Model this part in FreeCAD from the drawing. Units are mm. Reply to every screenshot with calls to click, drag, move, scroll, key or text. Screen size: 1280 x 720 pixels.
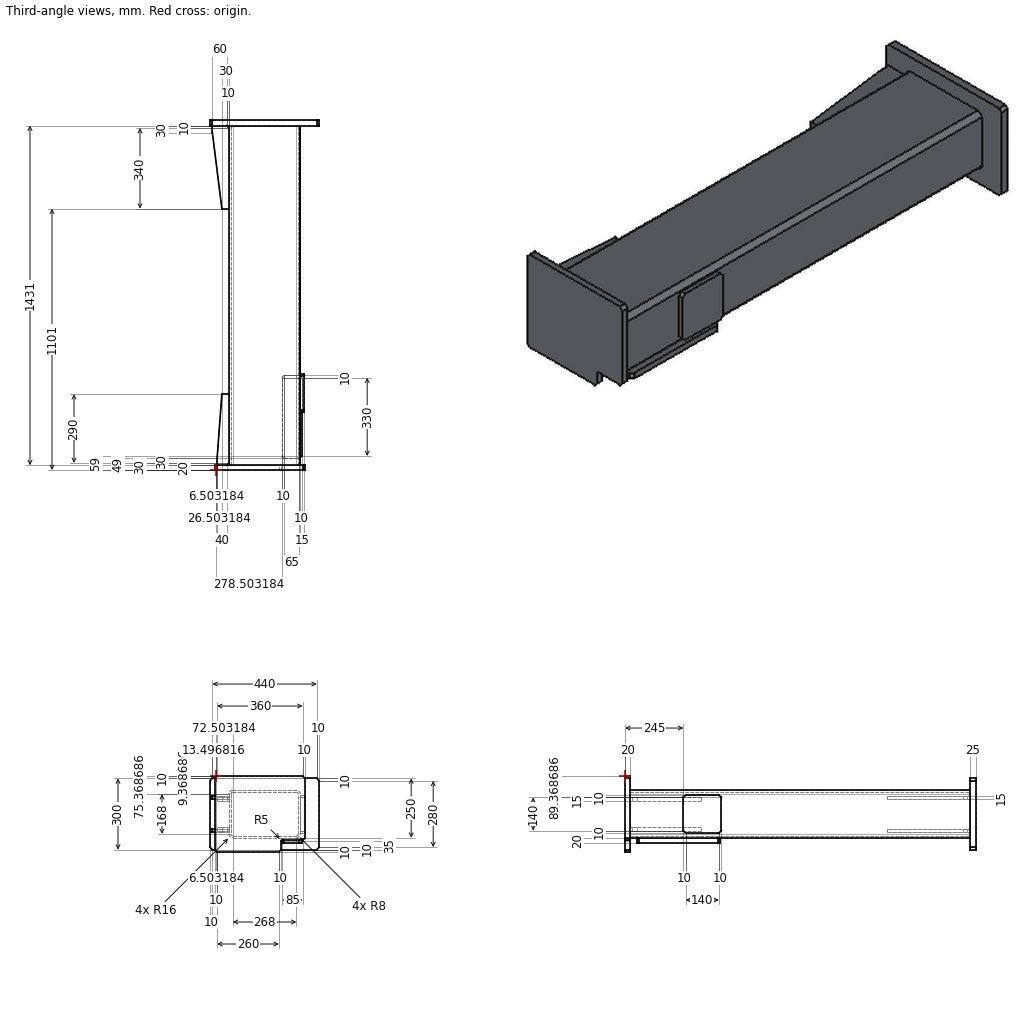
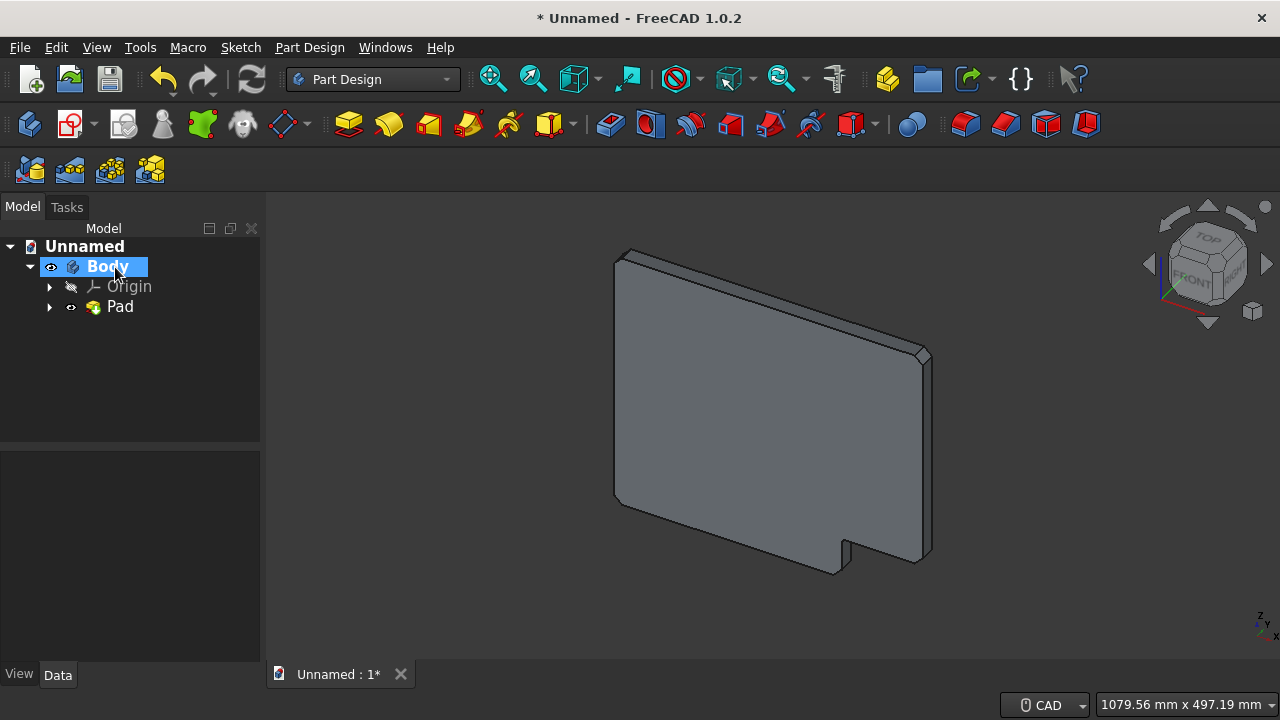
key(4)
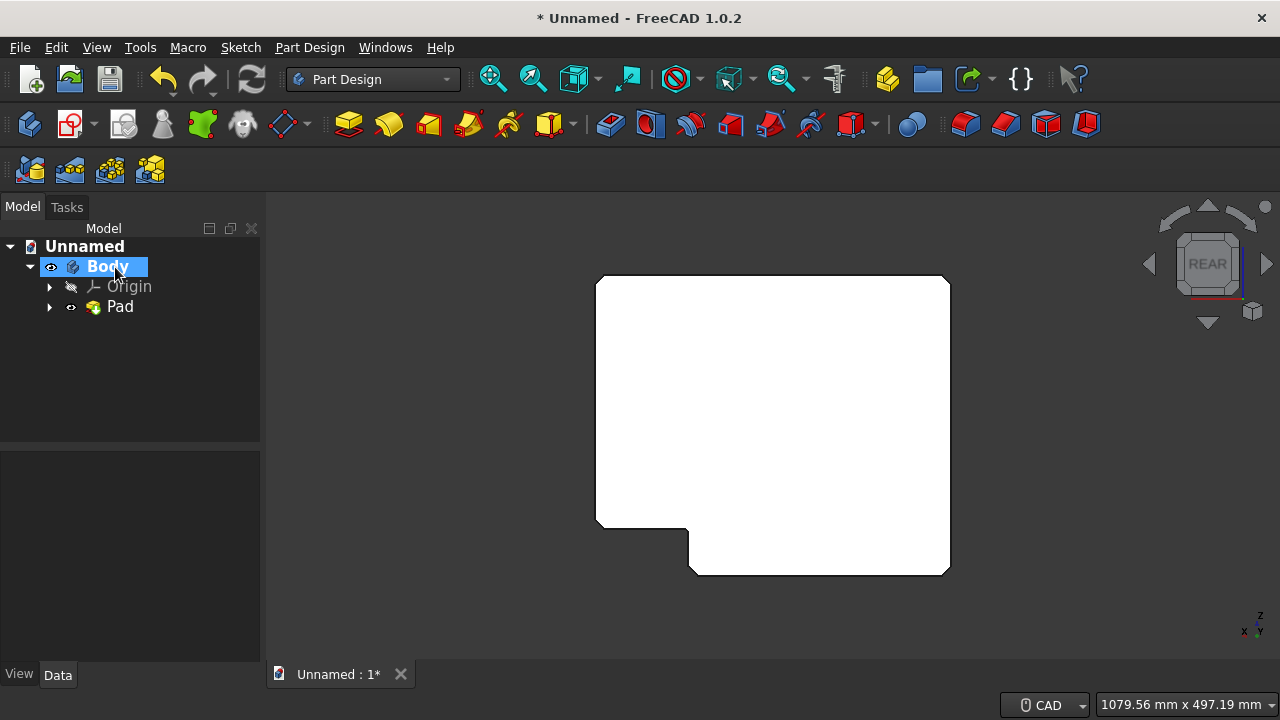
click(773, 424)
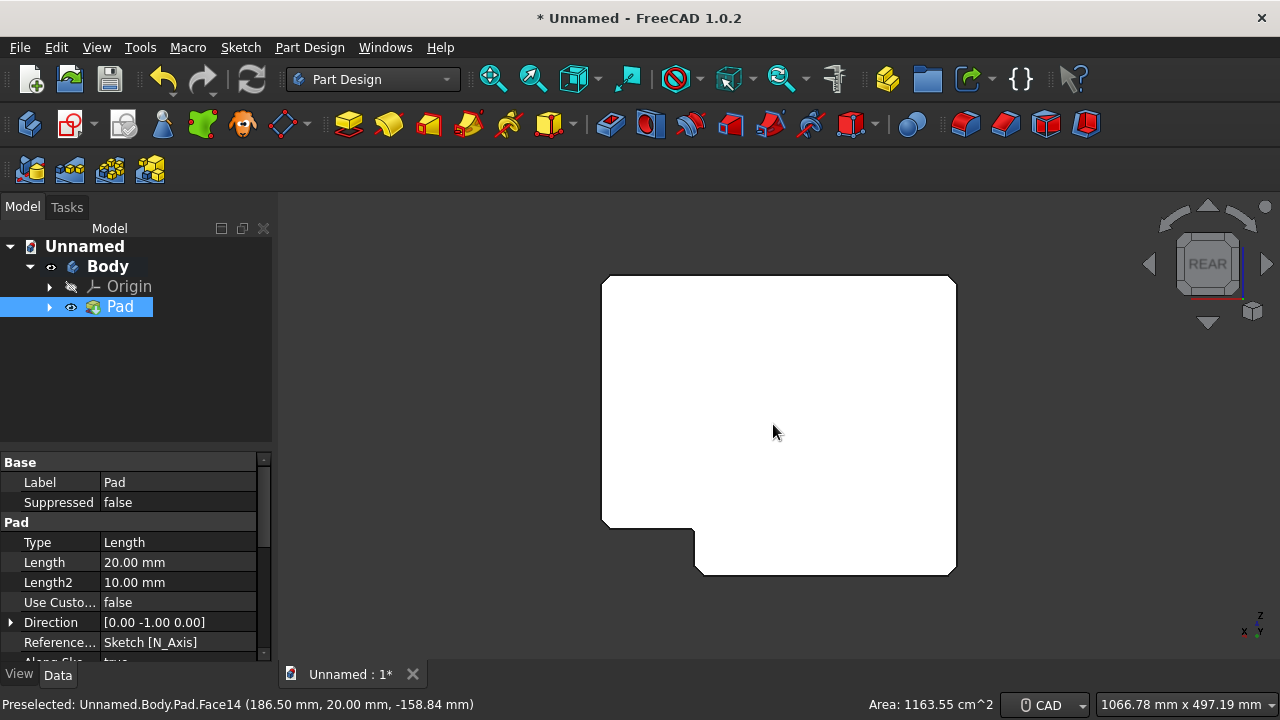
click(70, 124)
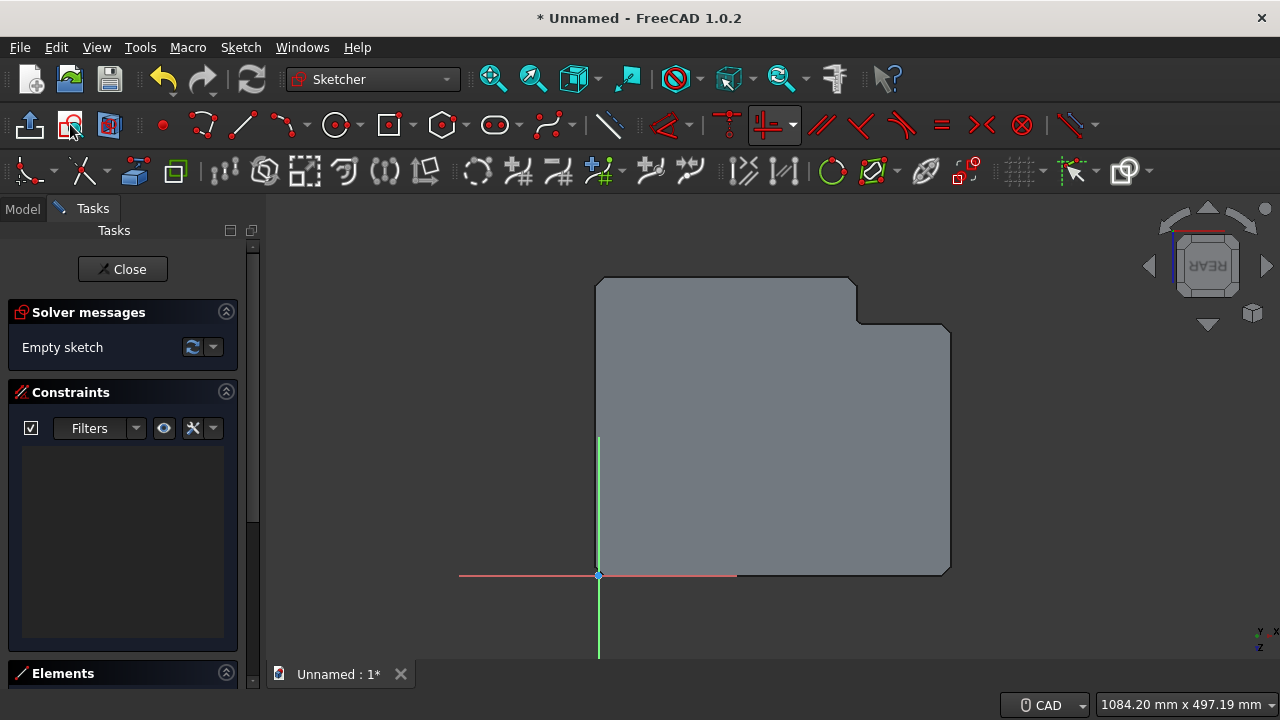
click(244, 126)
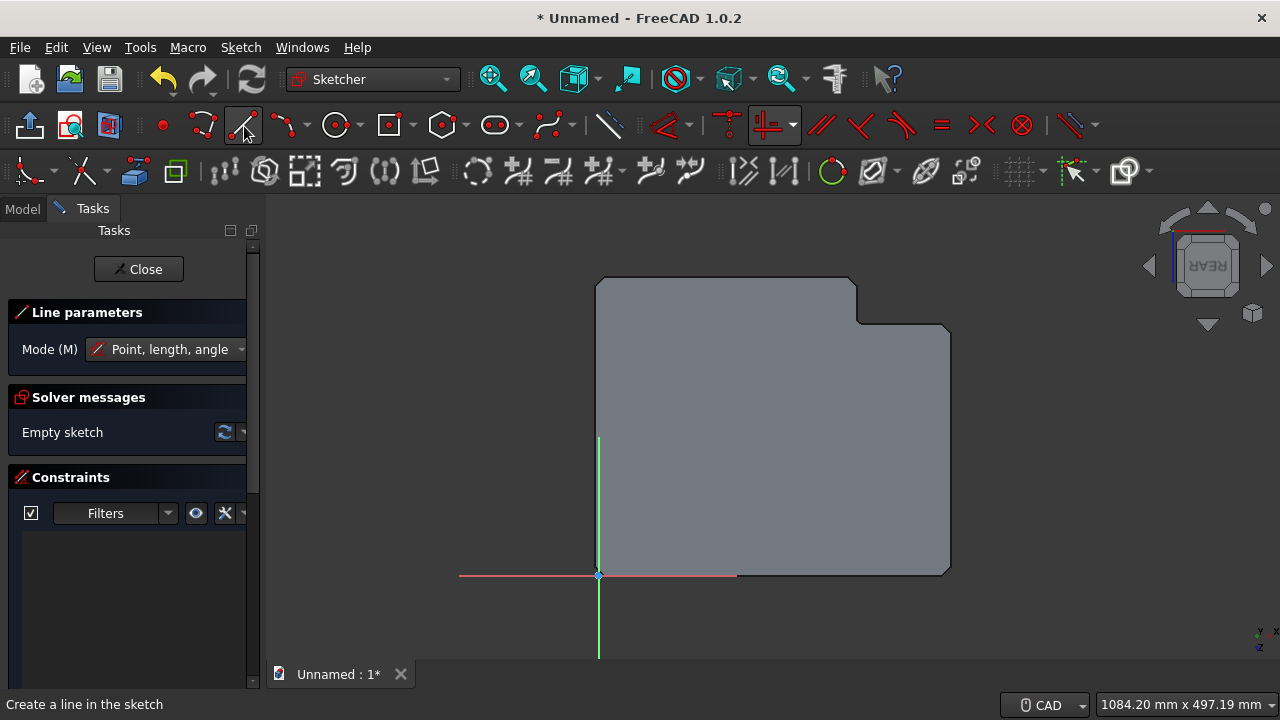
click(917, 333)
click(666, 333)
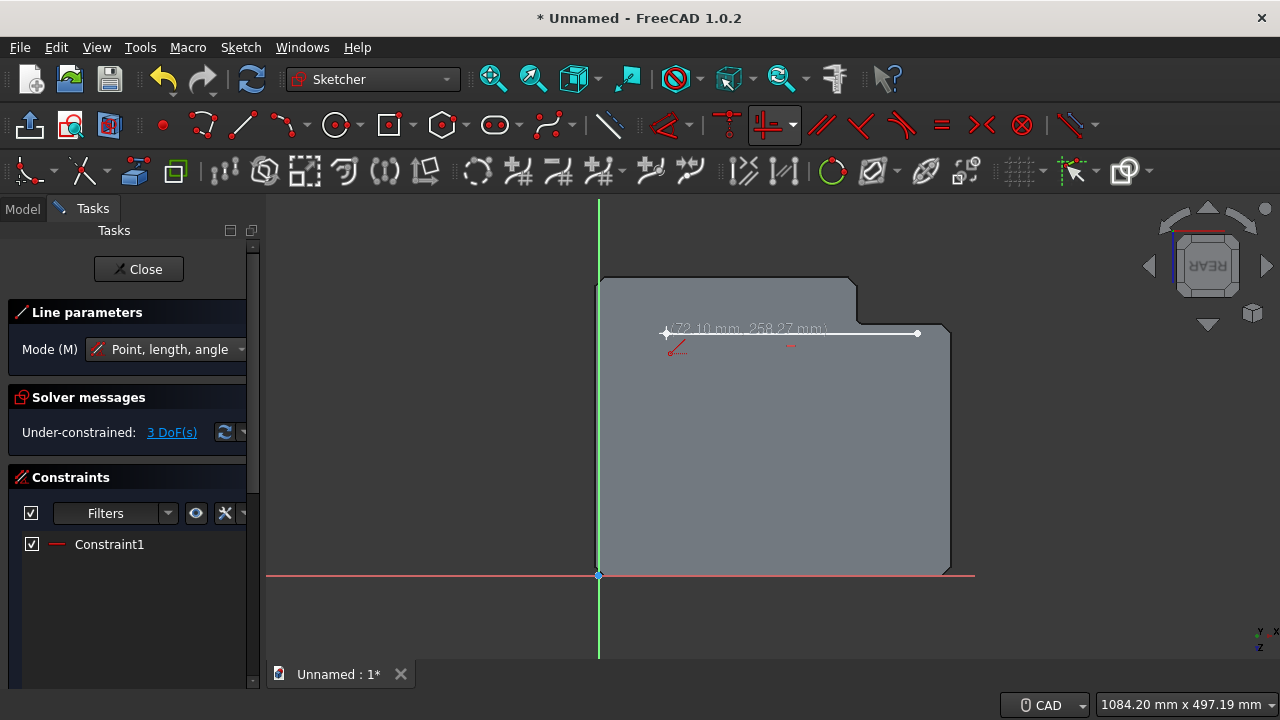
click(651, 348)
click(651, 505)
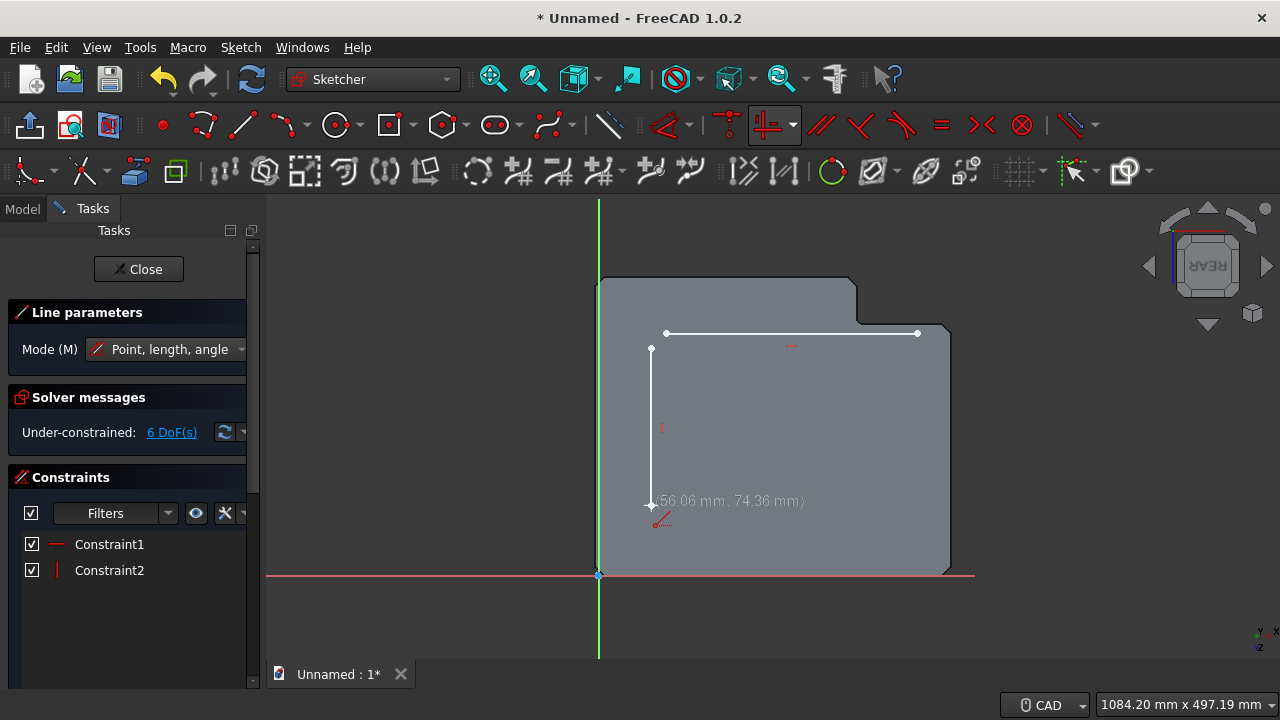
click(666, 520)
click(917, 520)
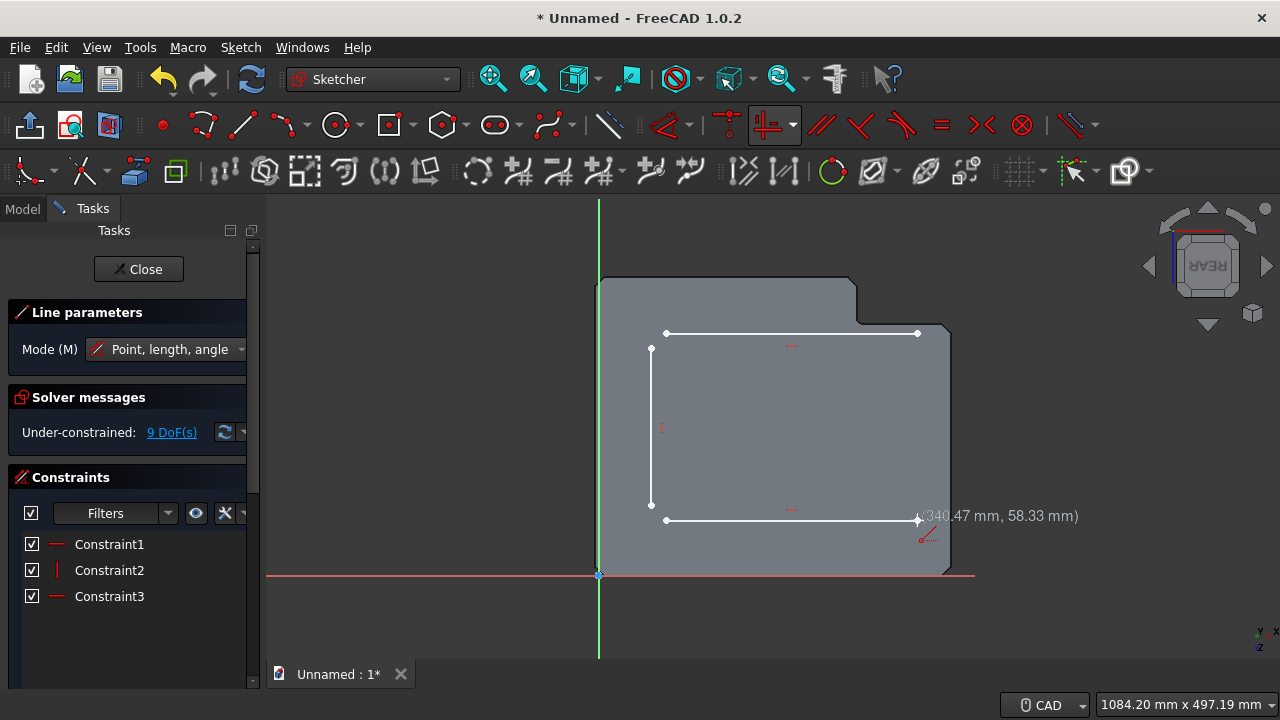
click(932, 505)
click(932, 348)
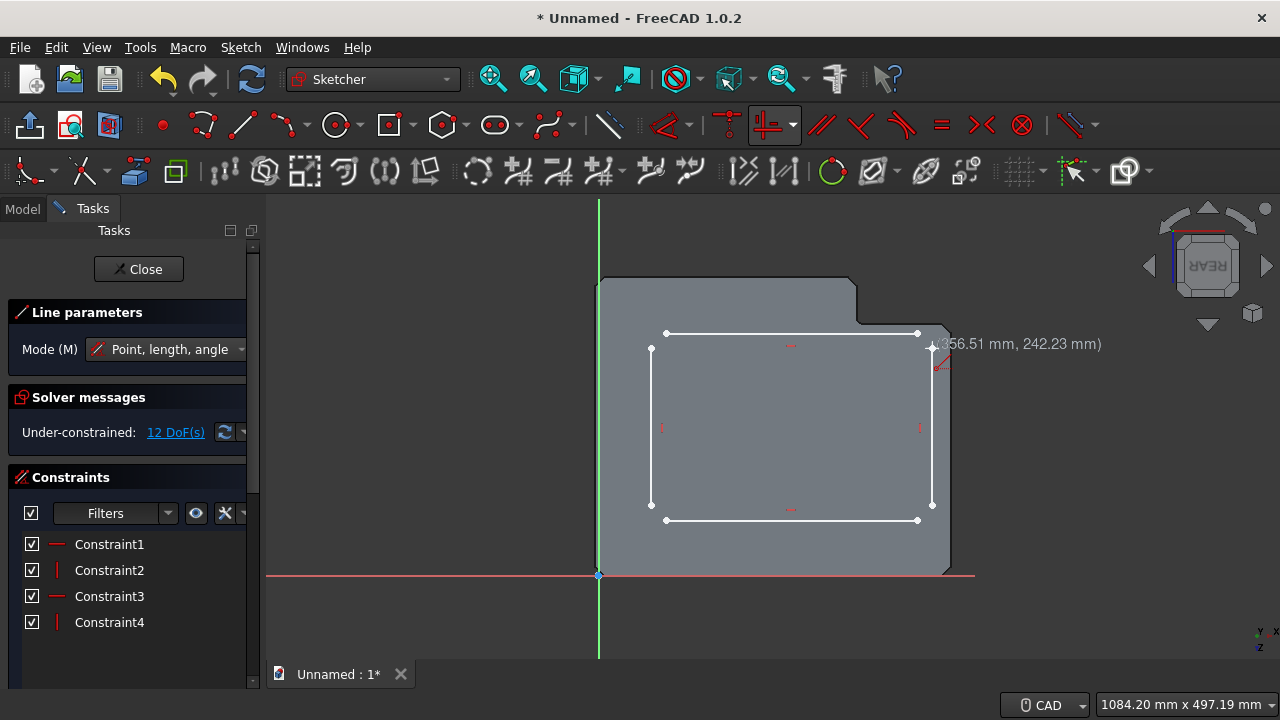
click(284, 126)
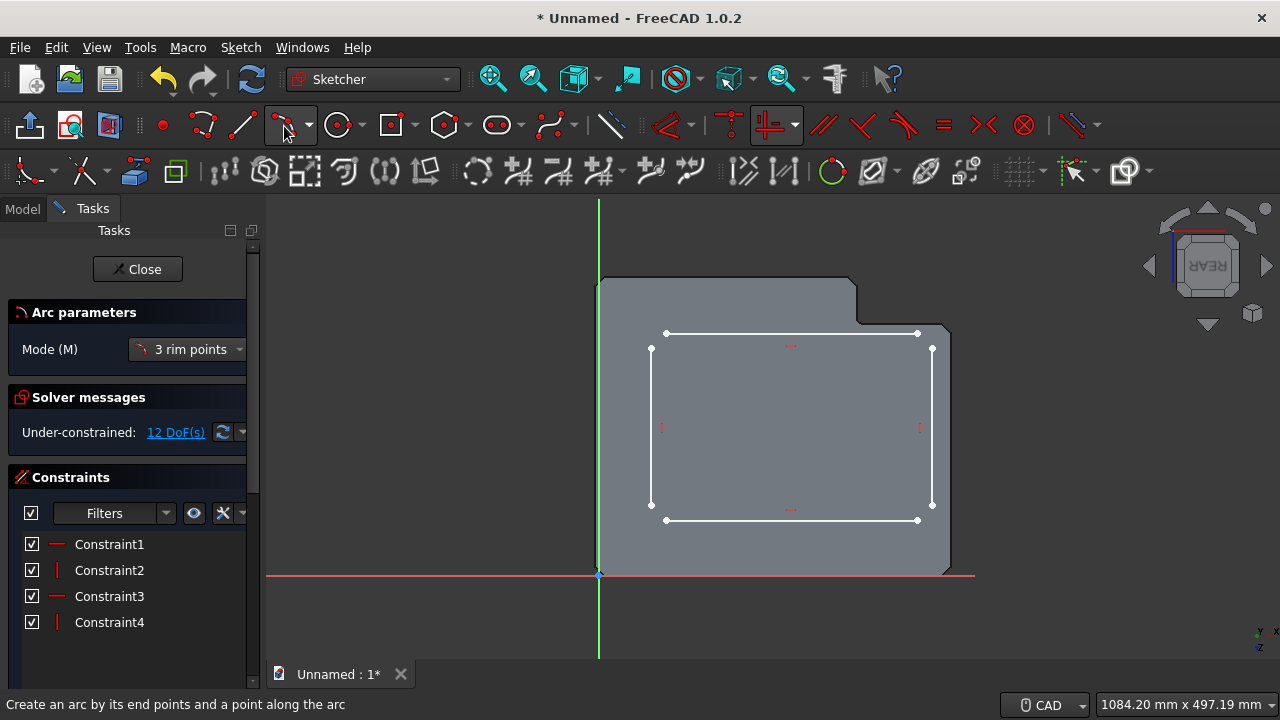
click(666, 334)
click(651, 349)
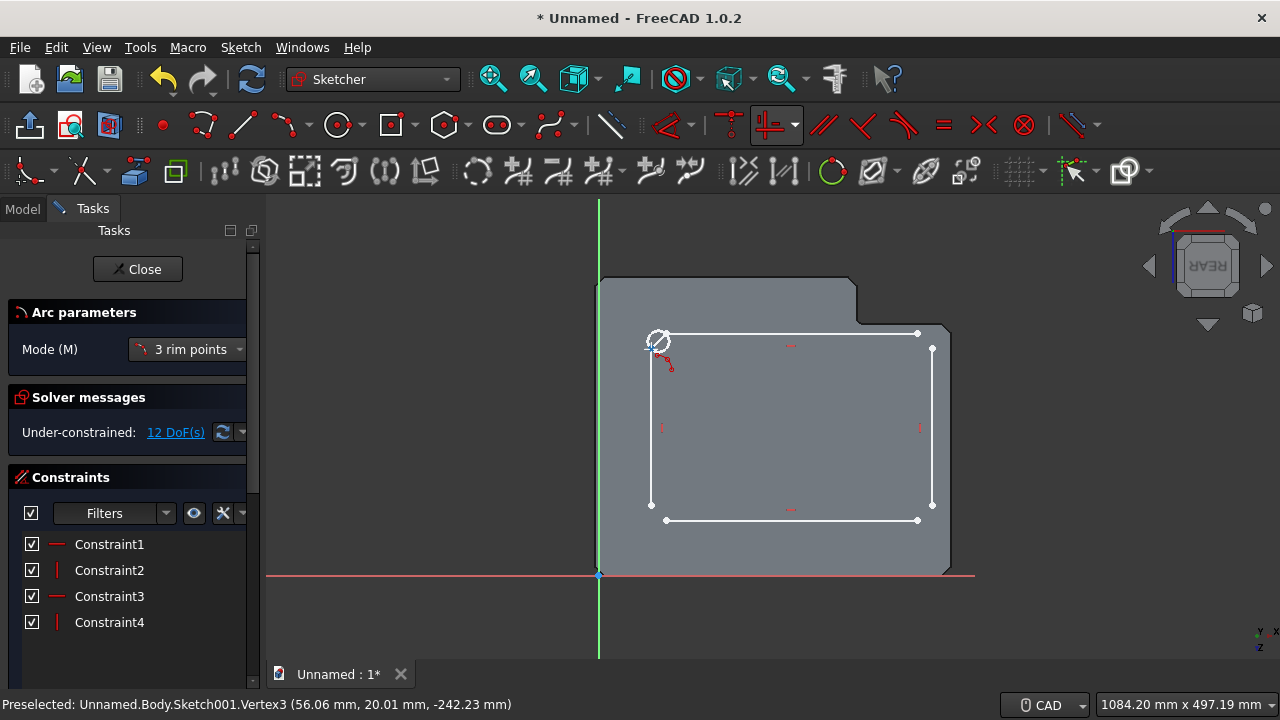
scroll(656, 337, up, 7)